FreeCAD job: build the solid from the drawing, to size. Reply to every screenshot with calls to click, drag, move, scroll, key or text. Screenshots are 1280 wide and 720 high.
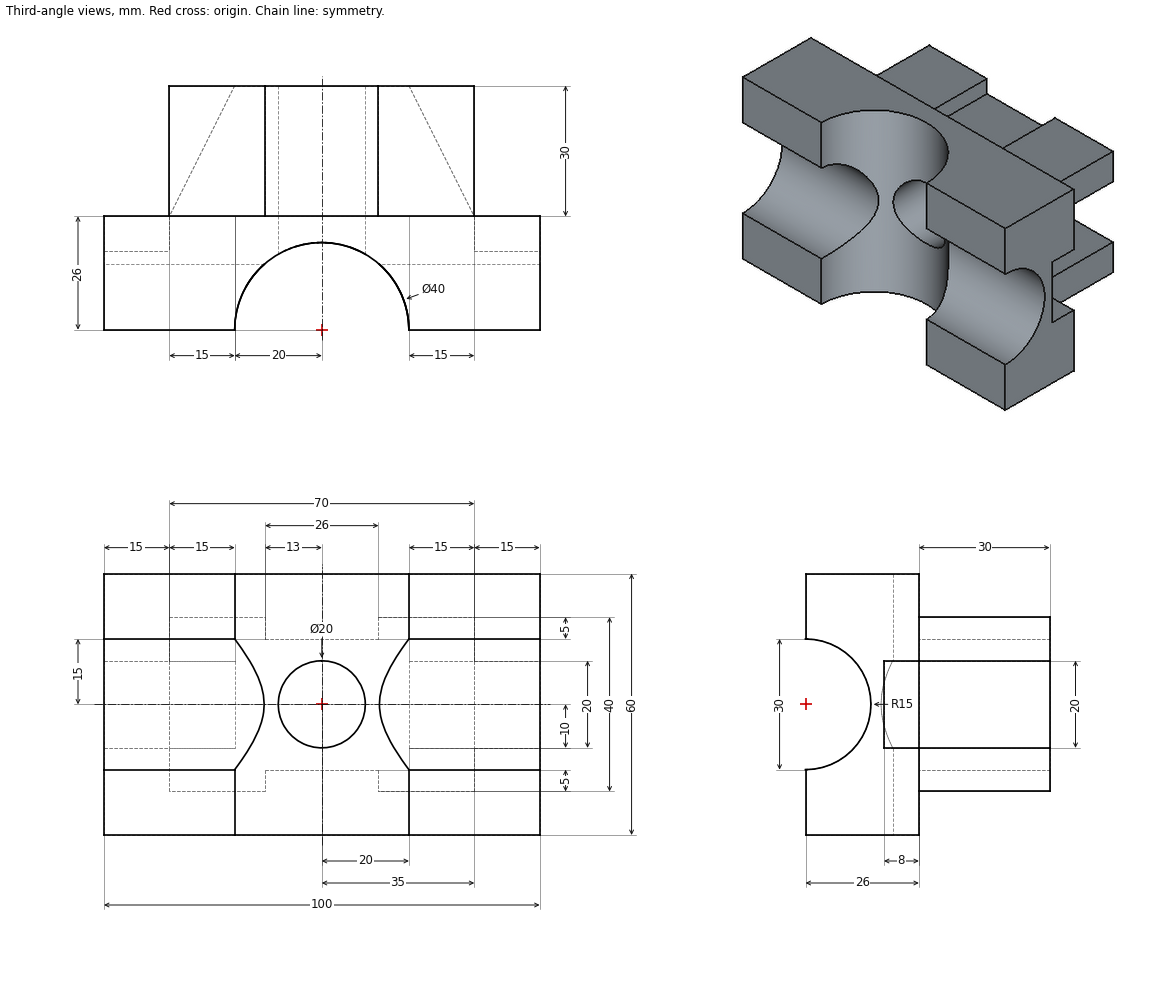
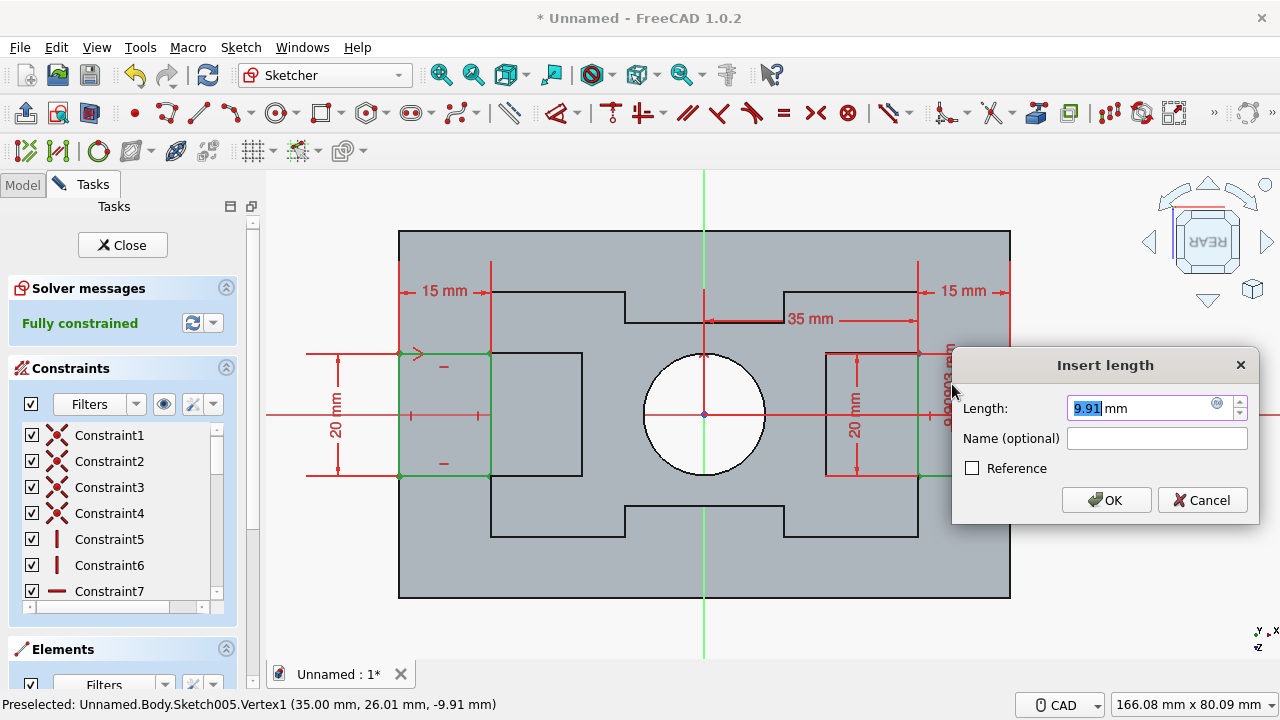
text(10)
key(Return)
key(Escape)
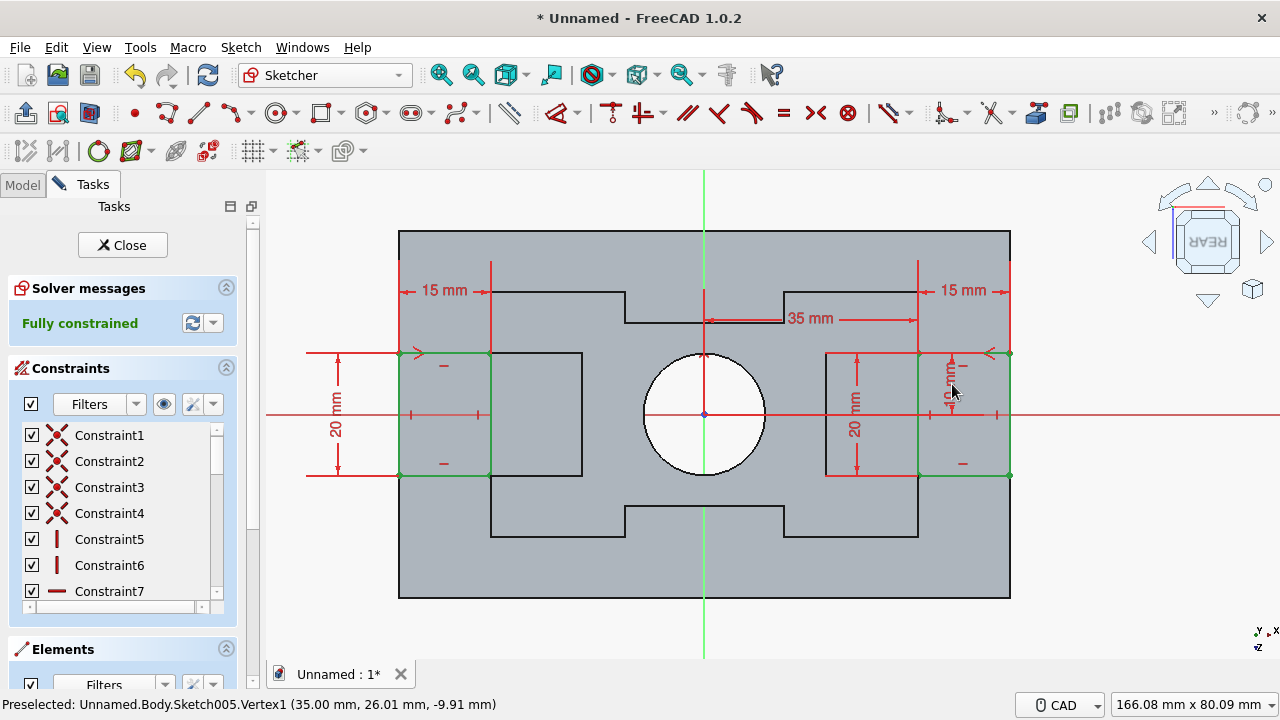
click(123, 245)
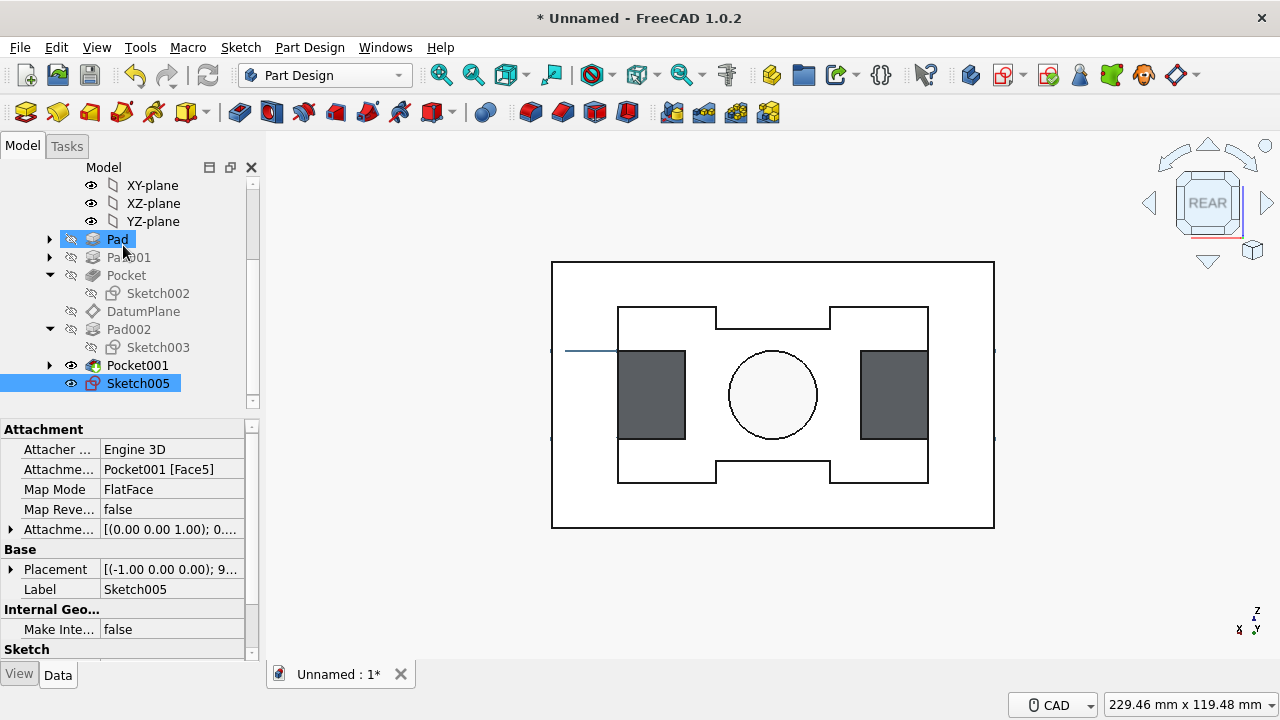
click(240, 112)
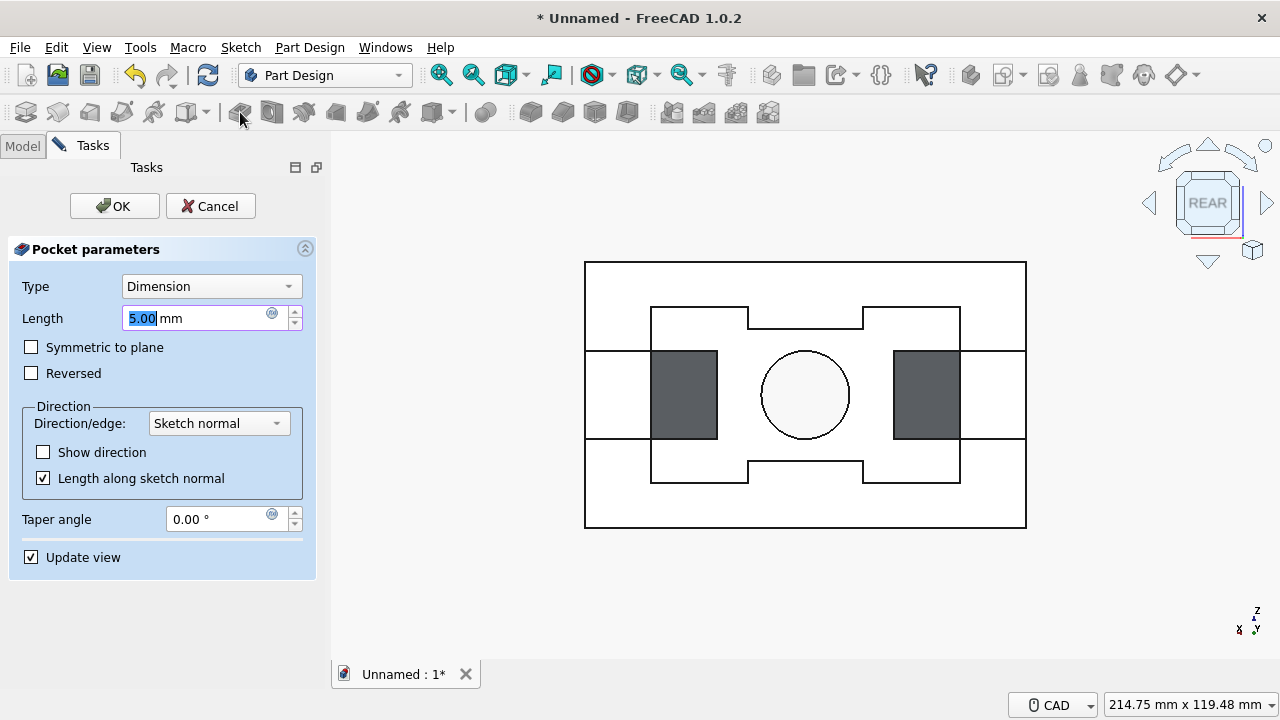
text(8)
key(Tab)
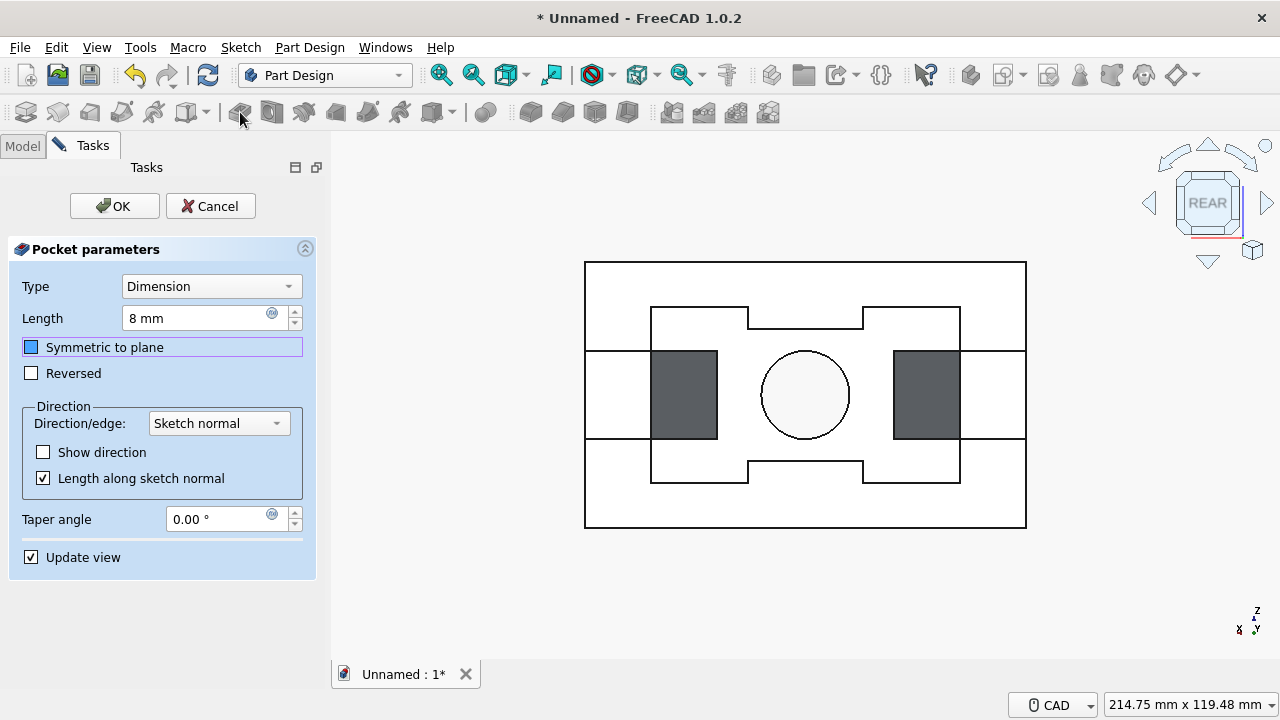
click(115, 206)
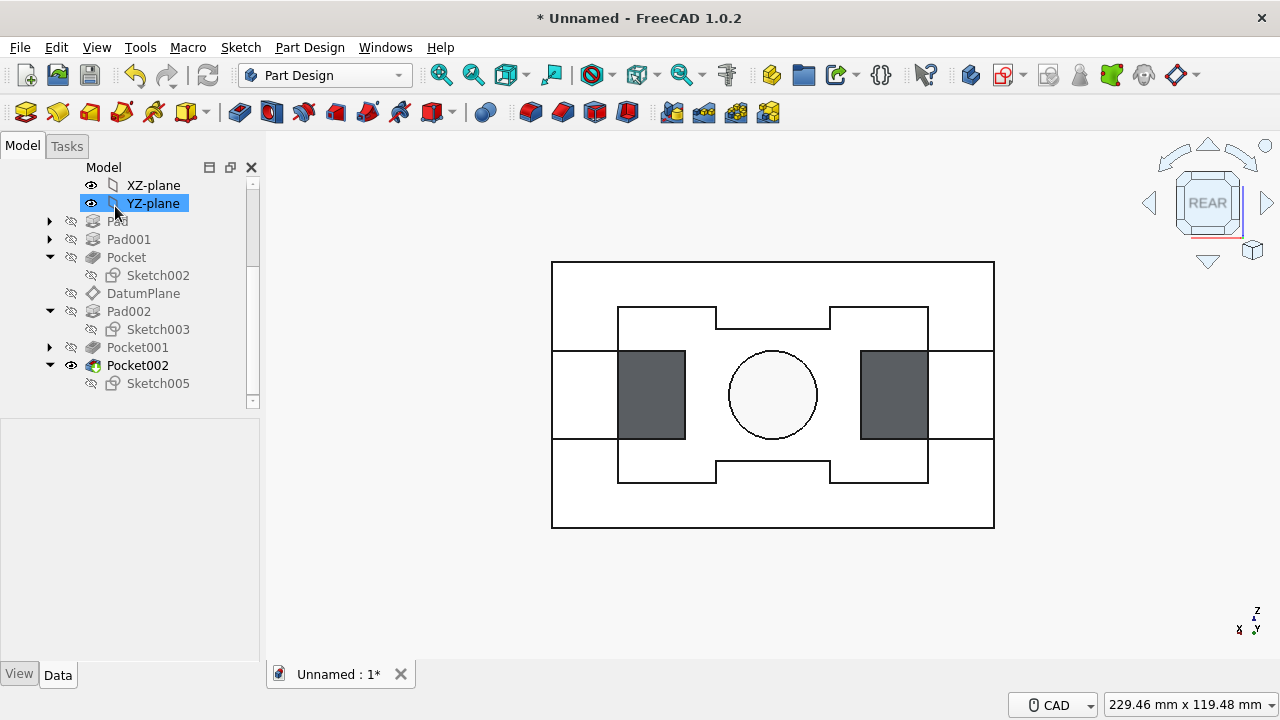
key(6)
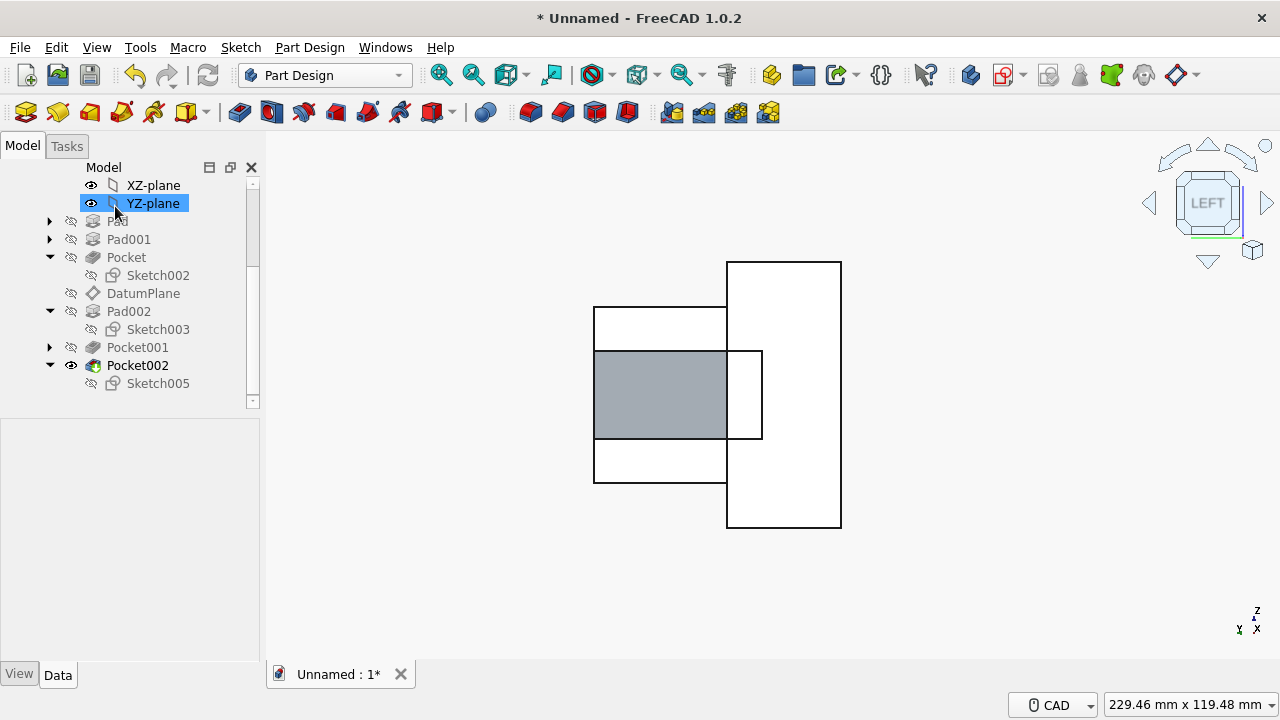
click(800, 318)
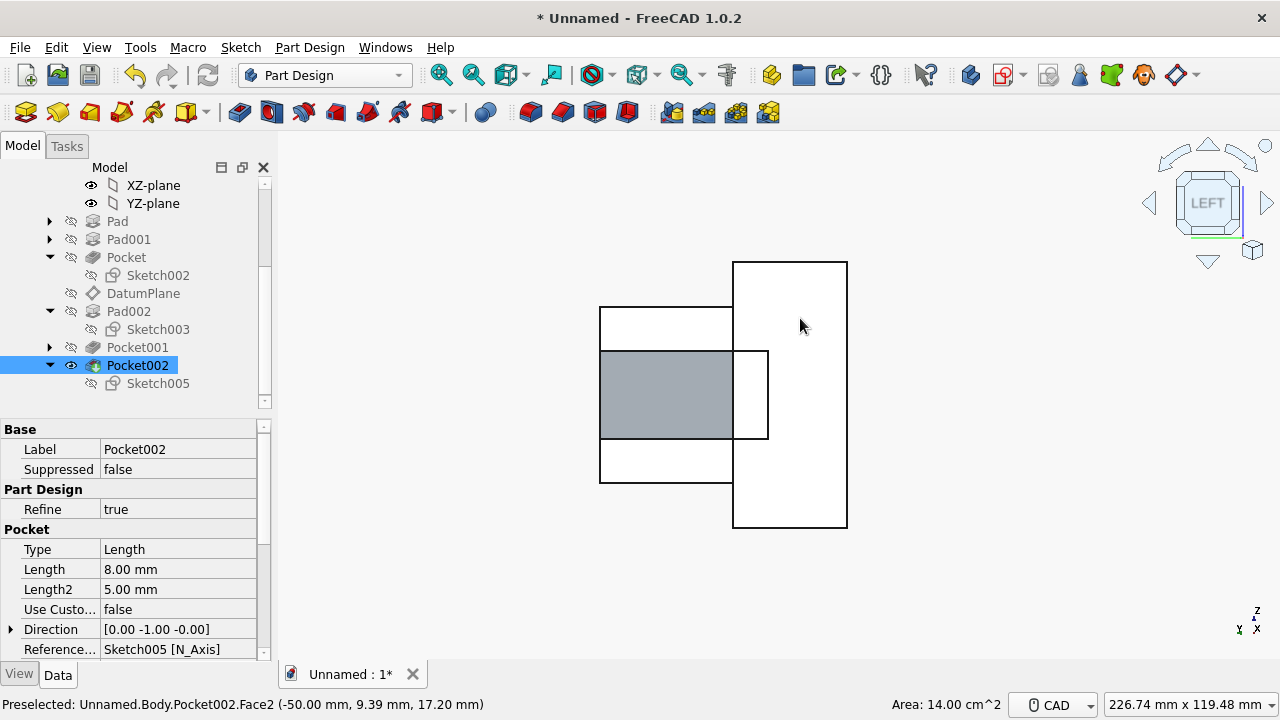
click(1004, 76)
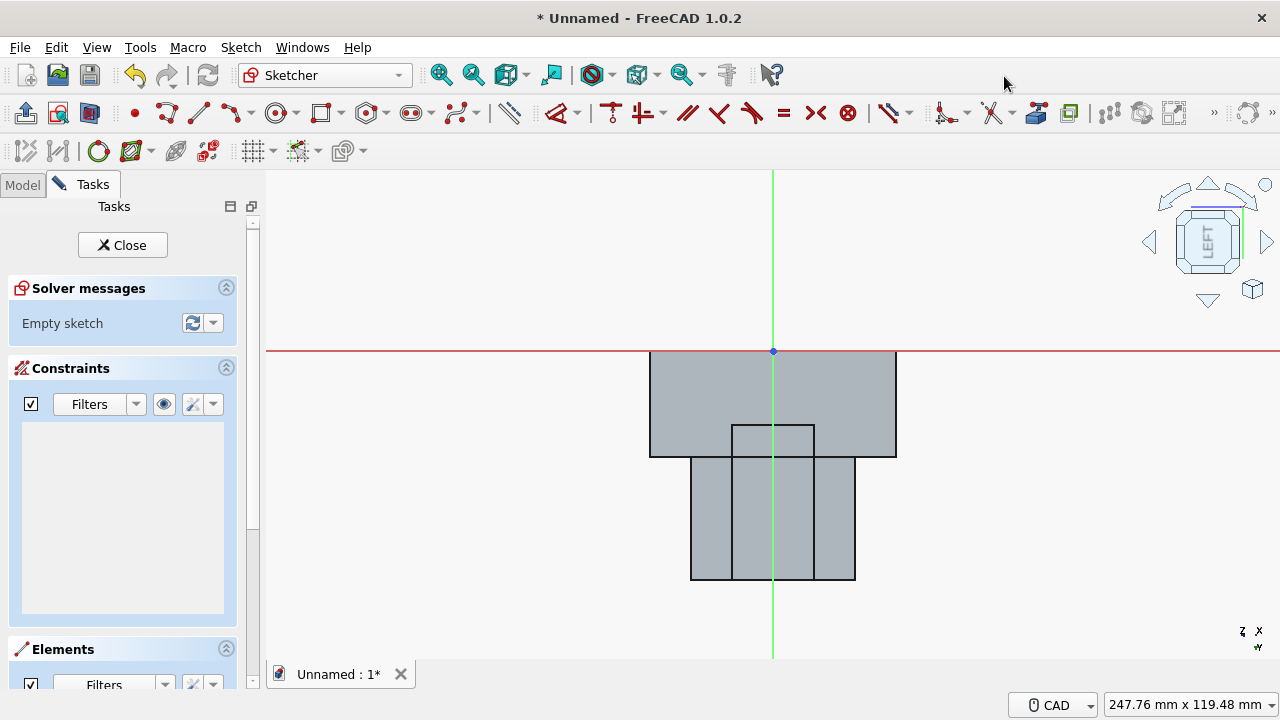
scroll(790, 373, up, 8)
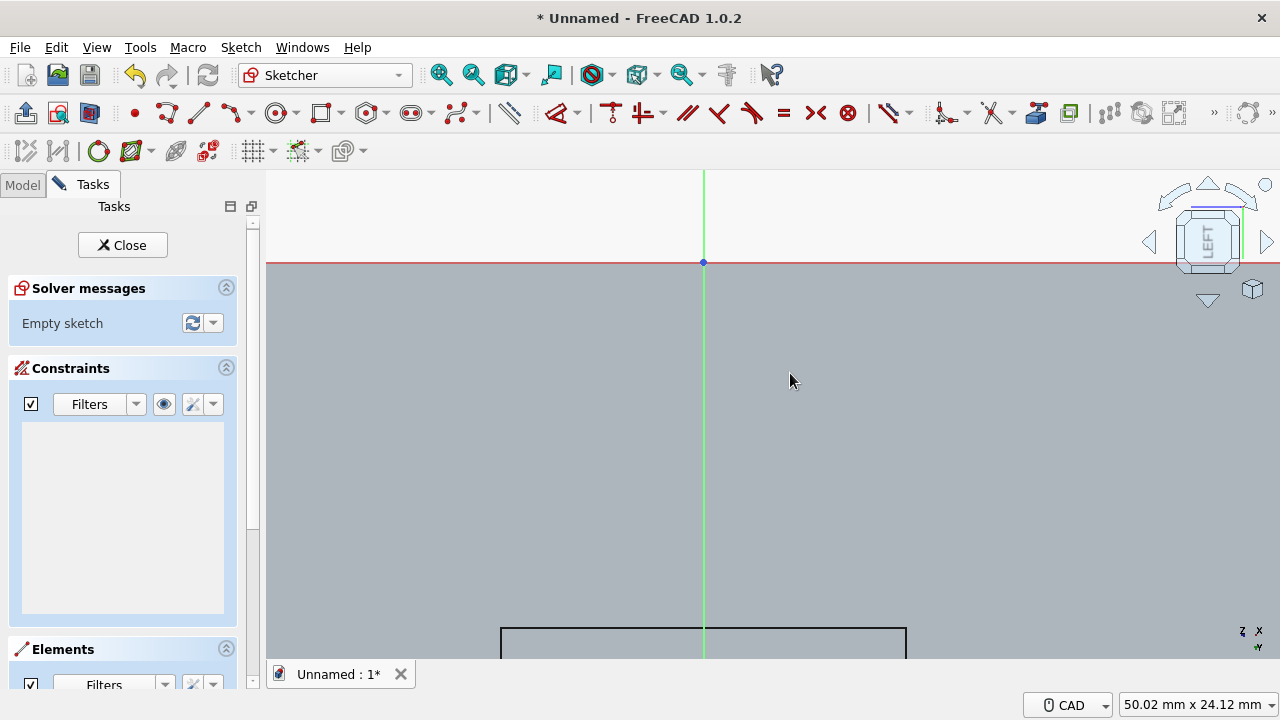
key(g)
key(l)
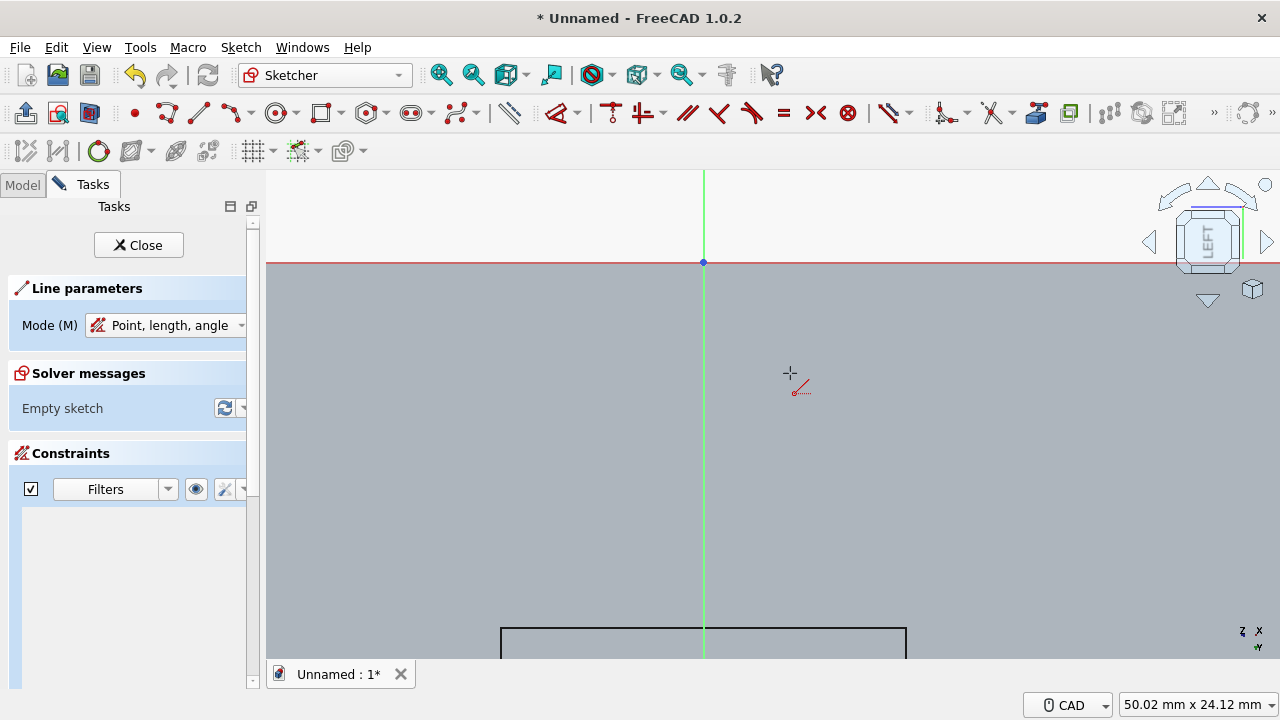
click(1008, 263)
click(400, 272)